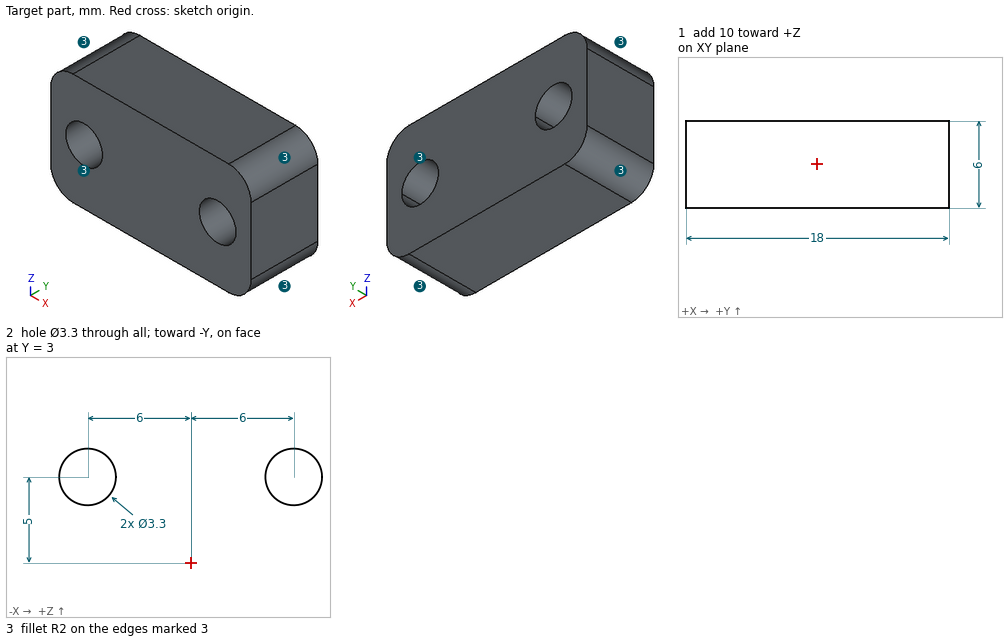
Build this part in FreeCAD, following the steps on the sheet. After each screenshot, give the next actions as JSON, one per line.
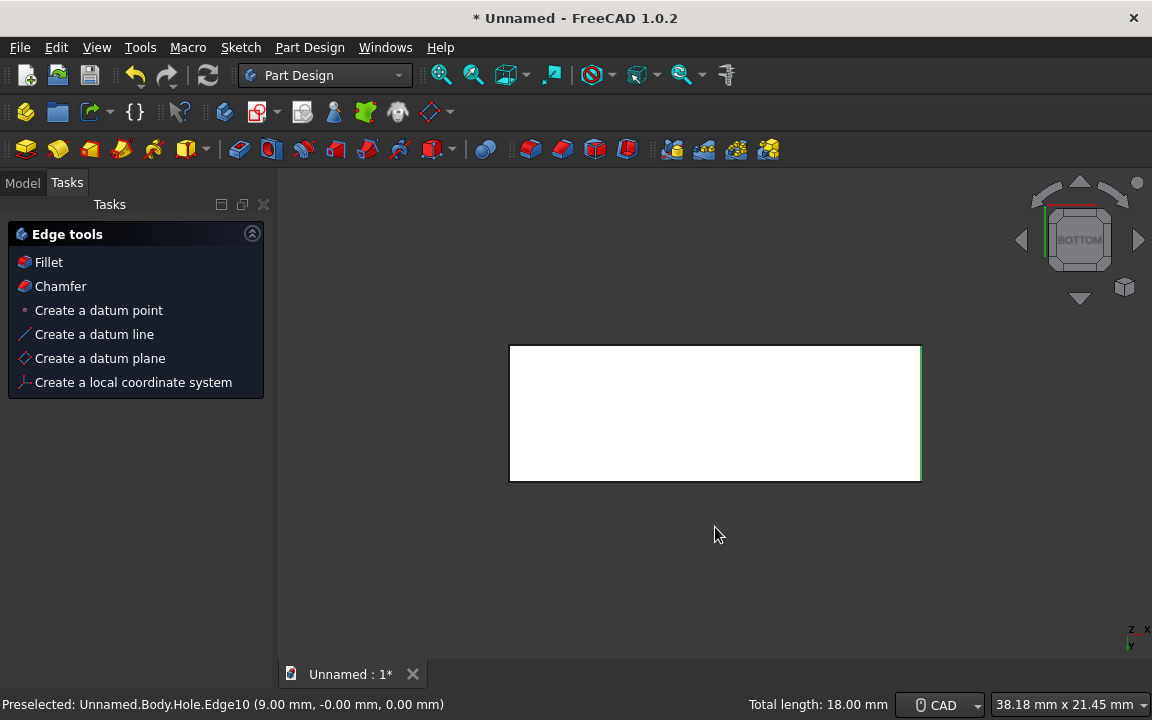
{"action": "left_click", "coordinate": [509, 413], "text": "ctrl"}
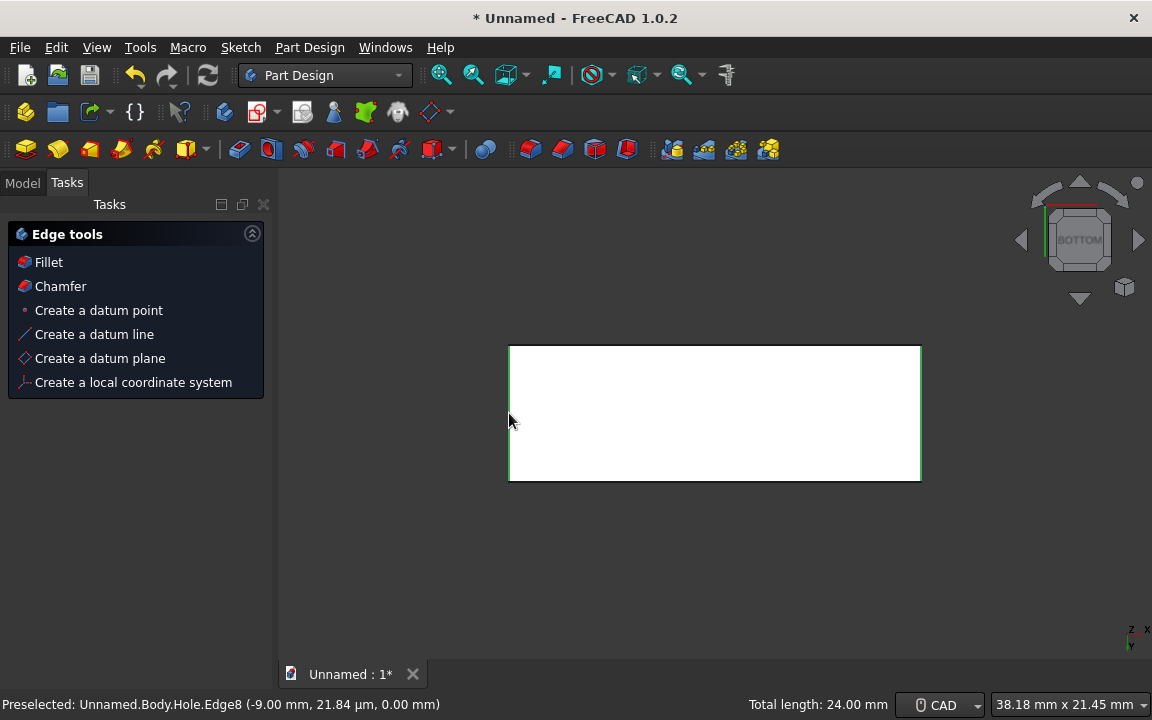
{"action": "left_click", "coordinate": [532, 150]}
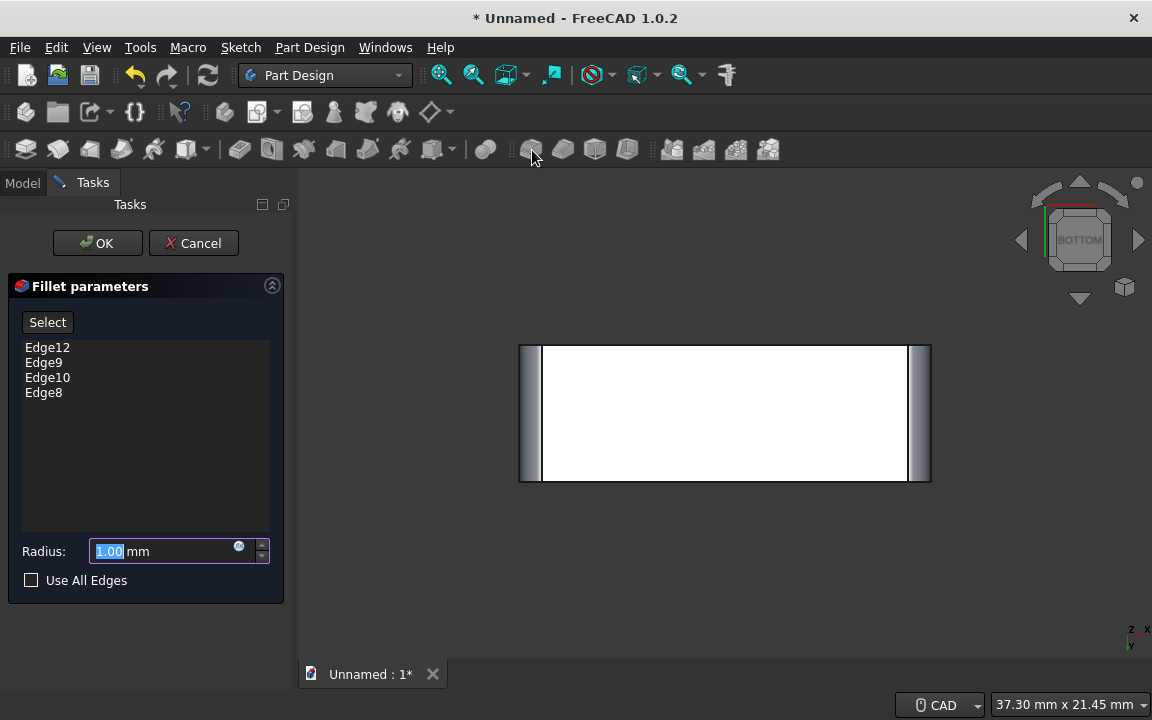
{"action": "type", "text": "2"}
{"action": "key", "text": "Tab"}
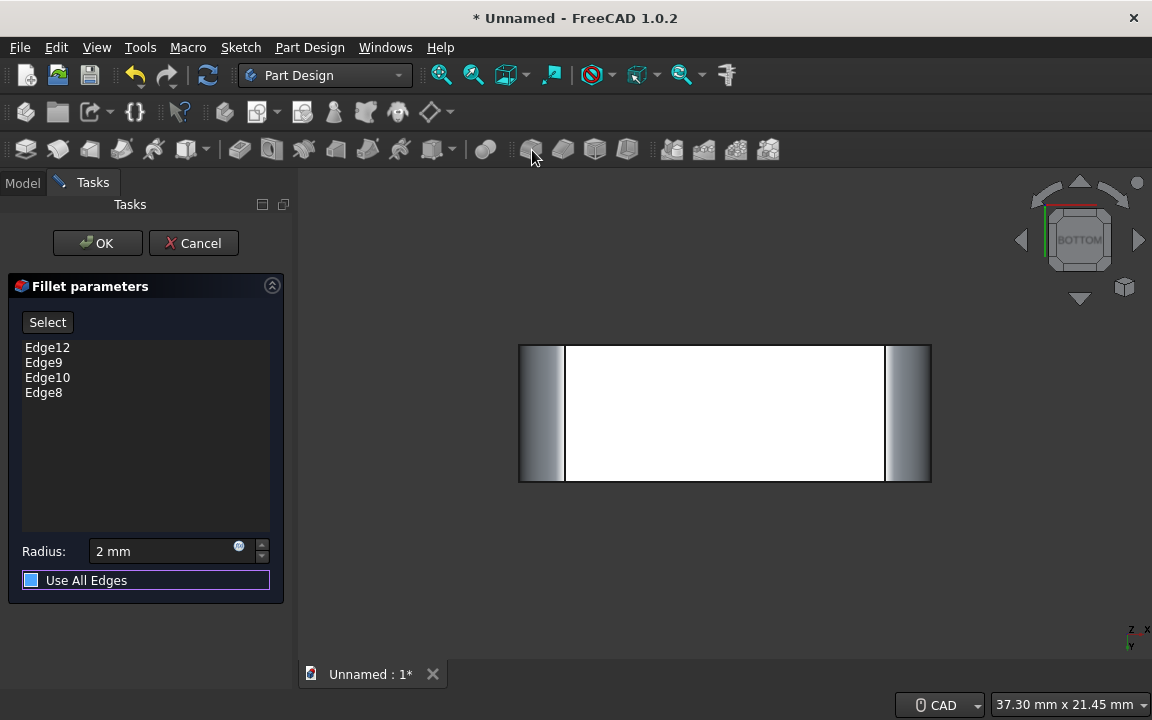
{"action": "left_click", "coordinate": [98, 243]}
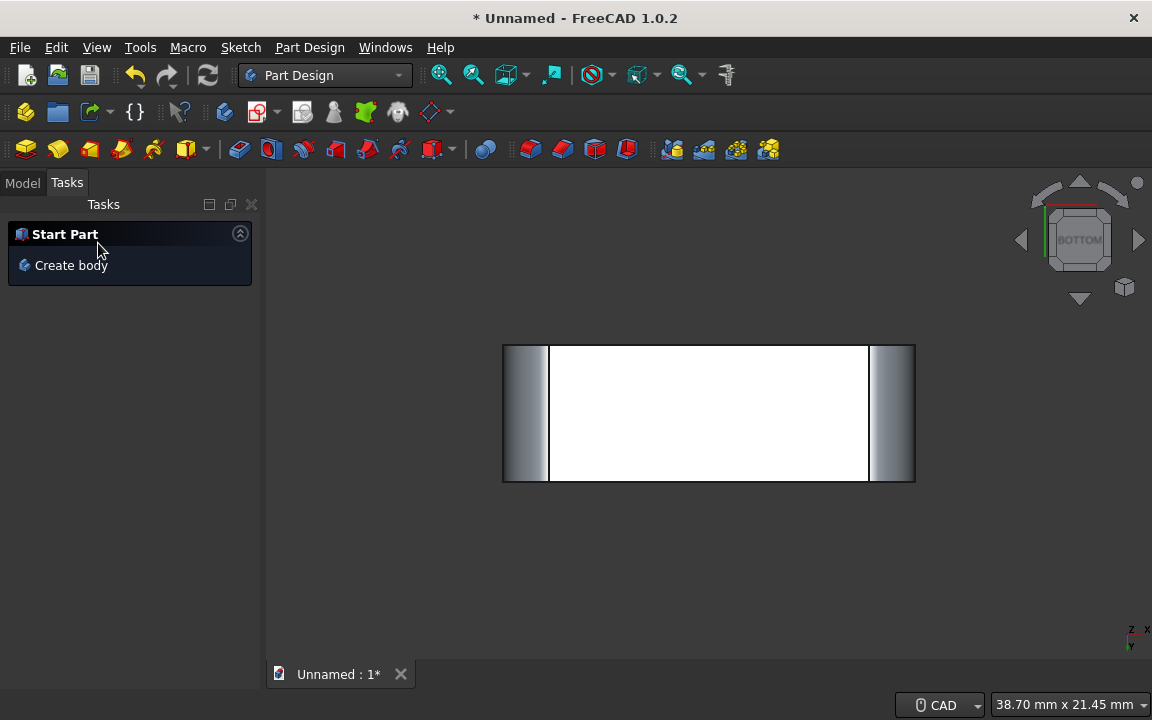
{"action": "key", "text": "0"}